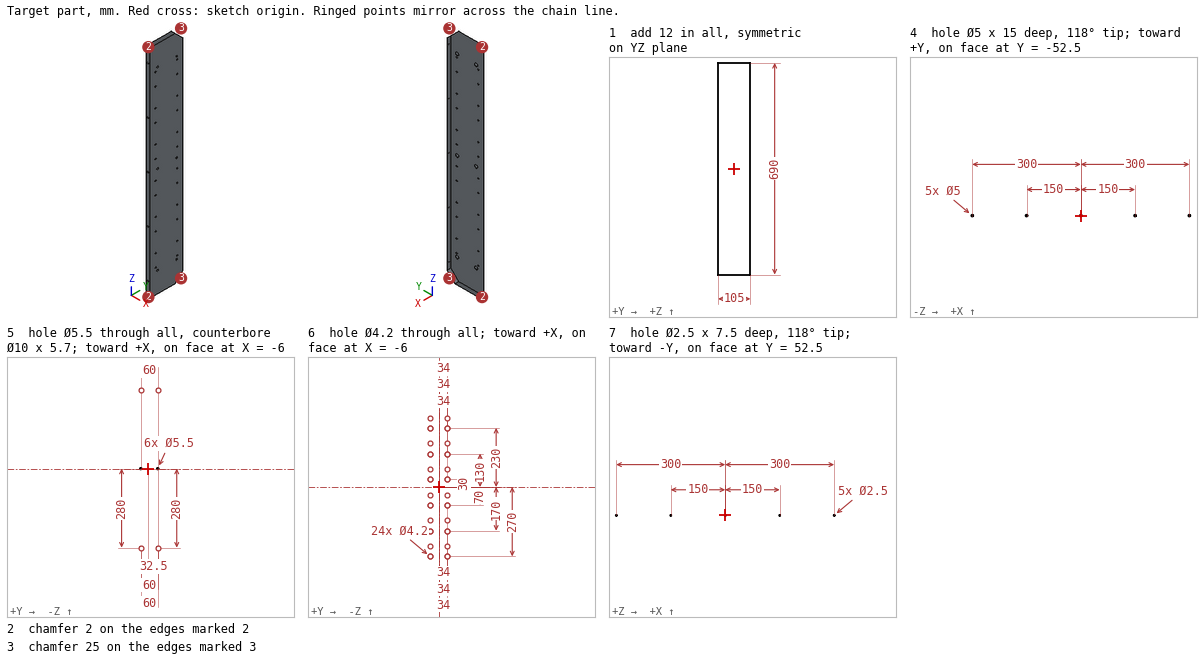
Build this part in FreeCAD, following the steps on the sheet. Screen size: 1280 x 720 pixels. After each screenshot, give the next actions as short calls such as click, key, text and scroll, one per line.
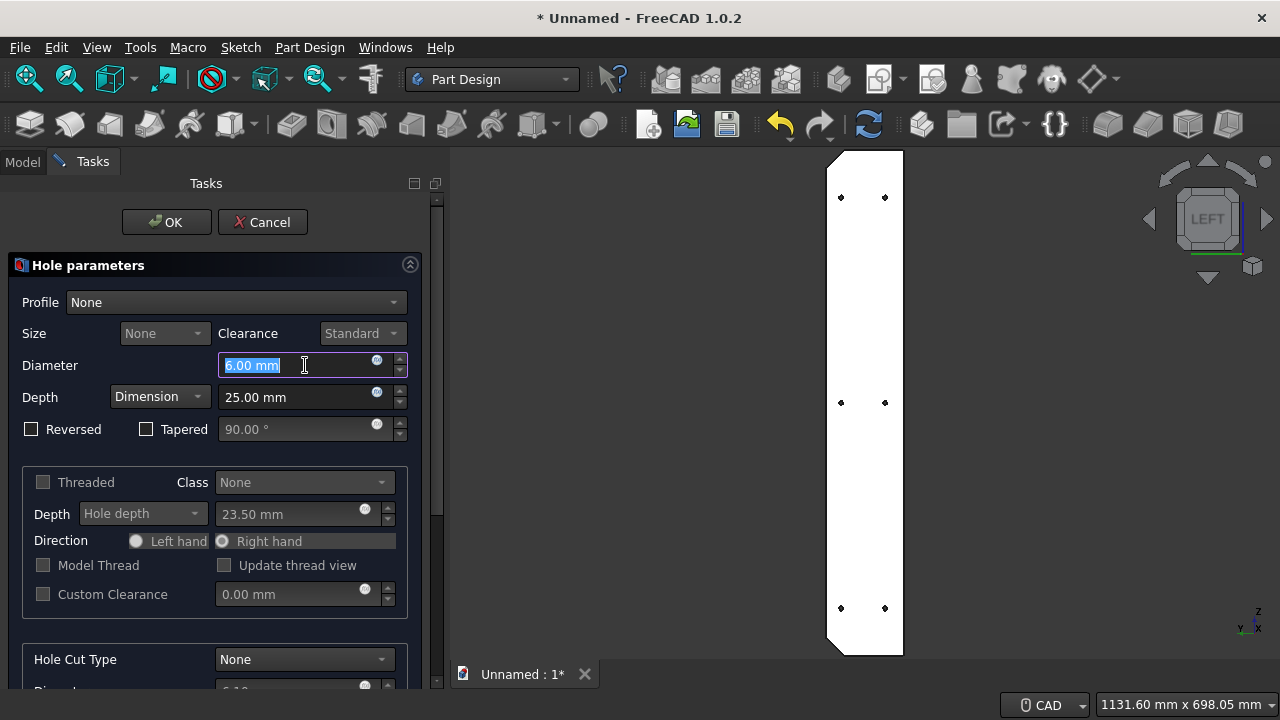
text(5.5)
key(Tab)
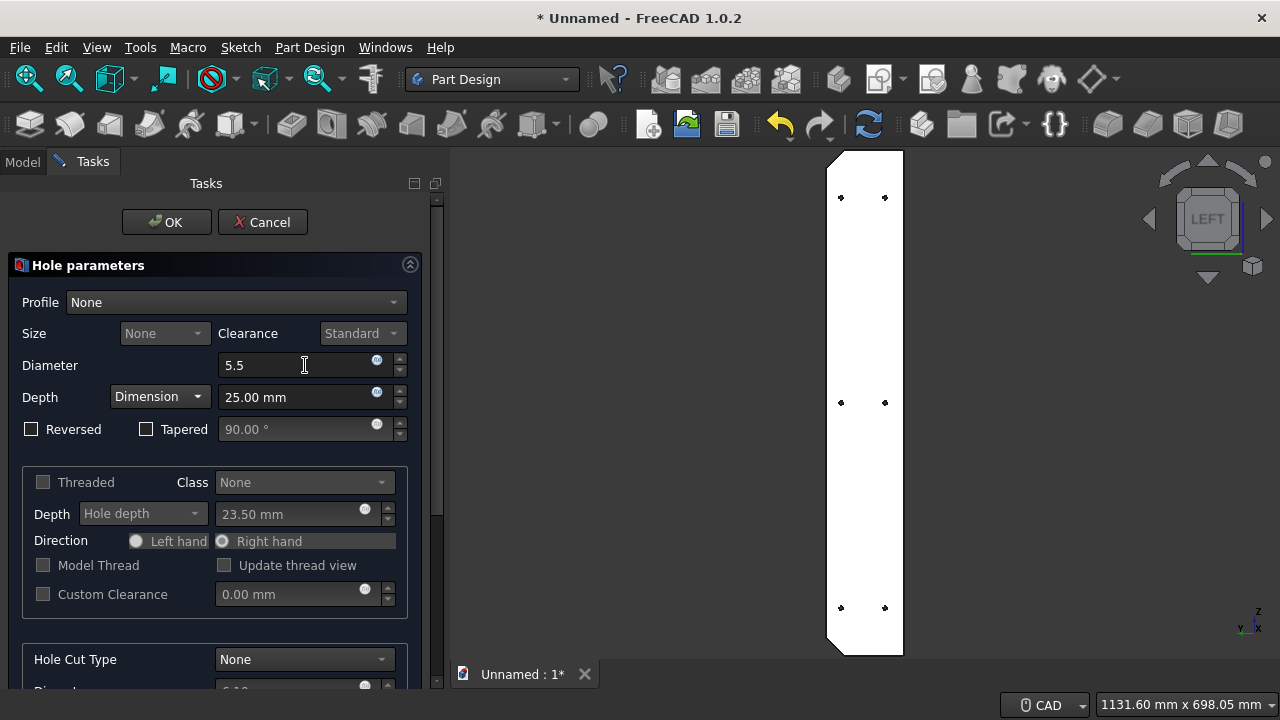
click(161, 396)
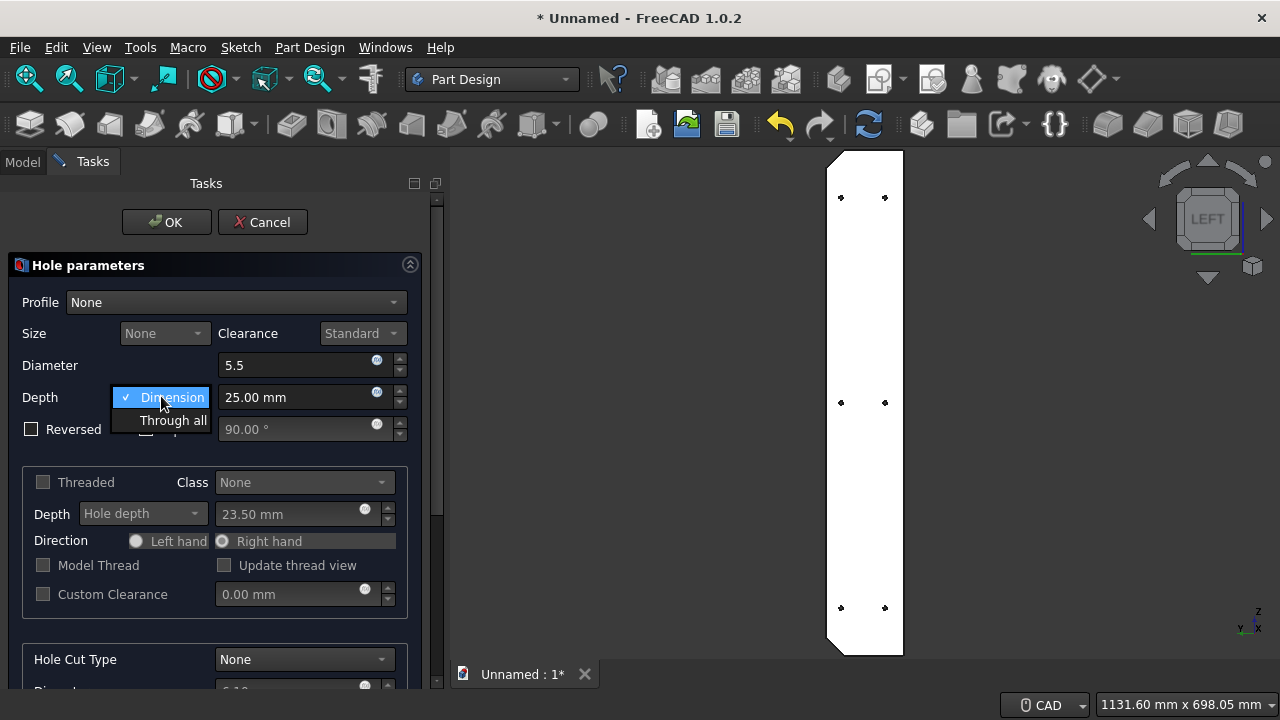
click(160, 420)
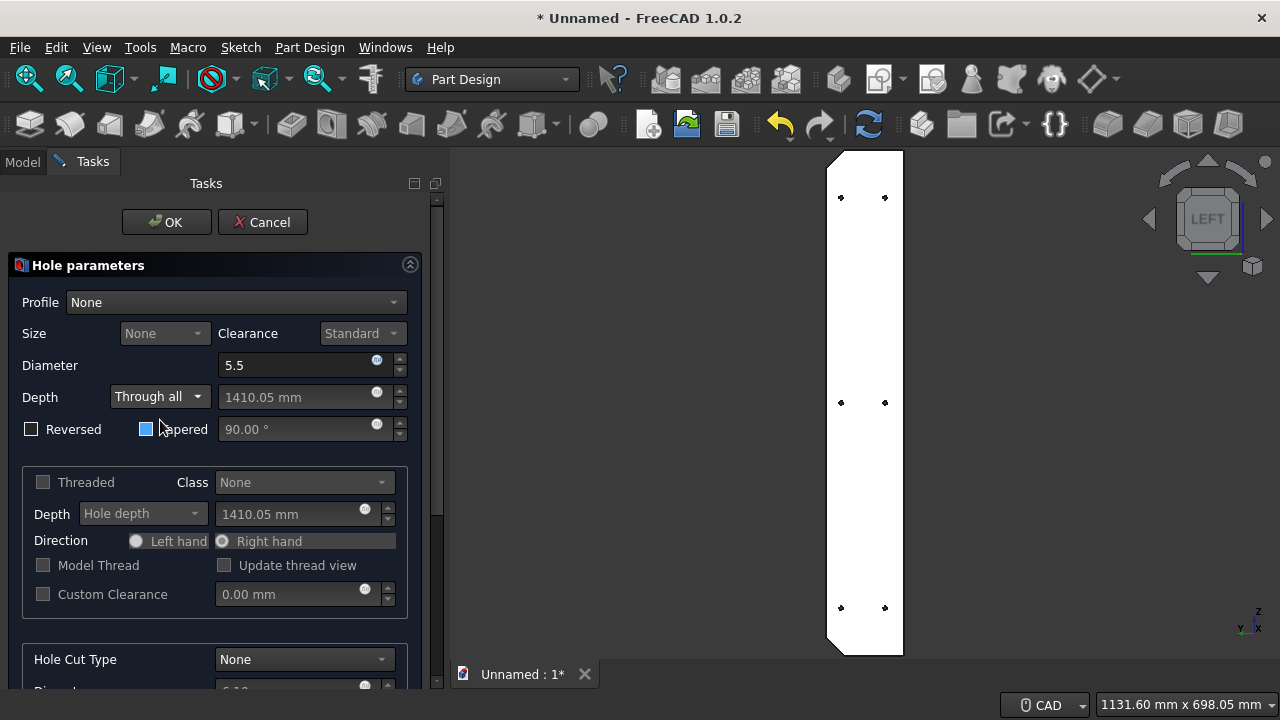
click(306, 660)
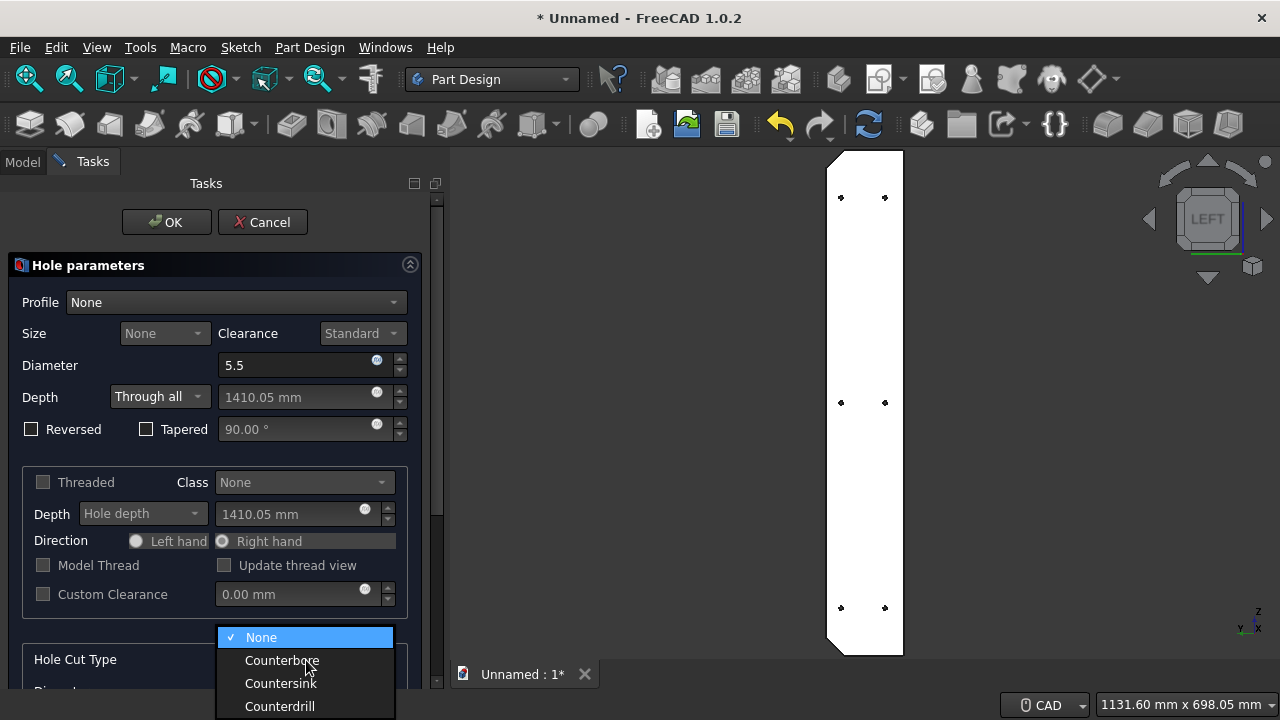
click(304, 660)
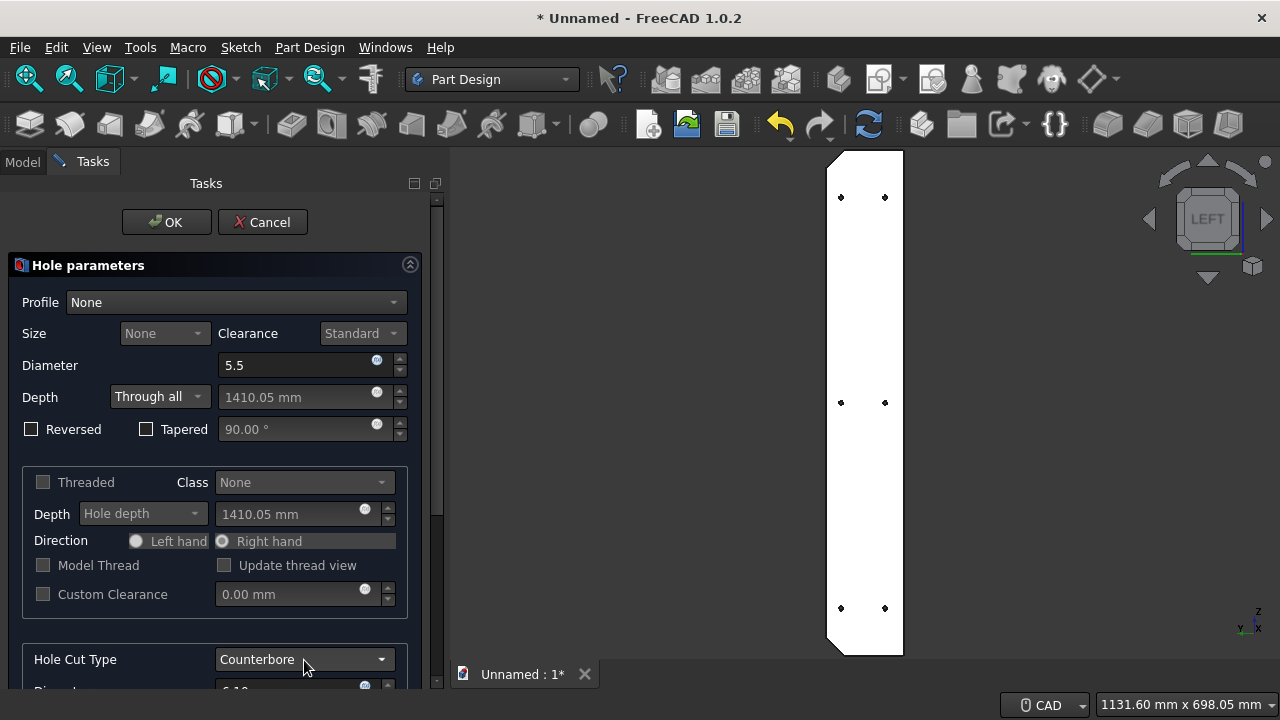
scroll(437, 440, down, 2)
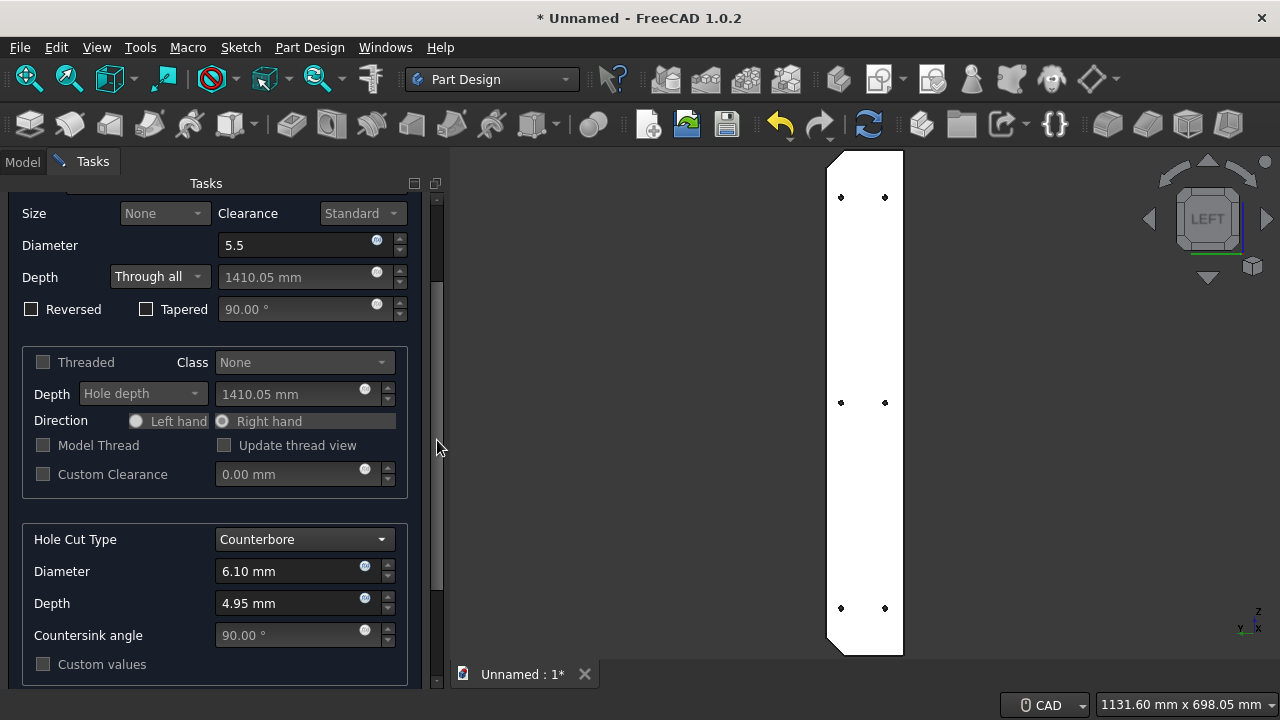
triple_click(298, 571)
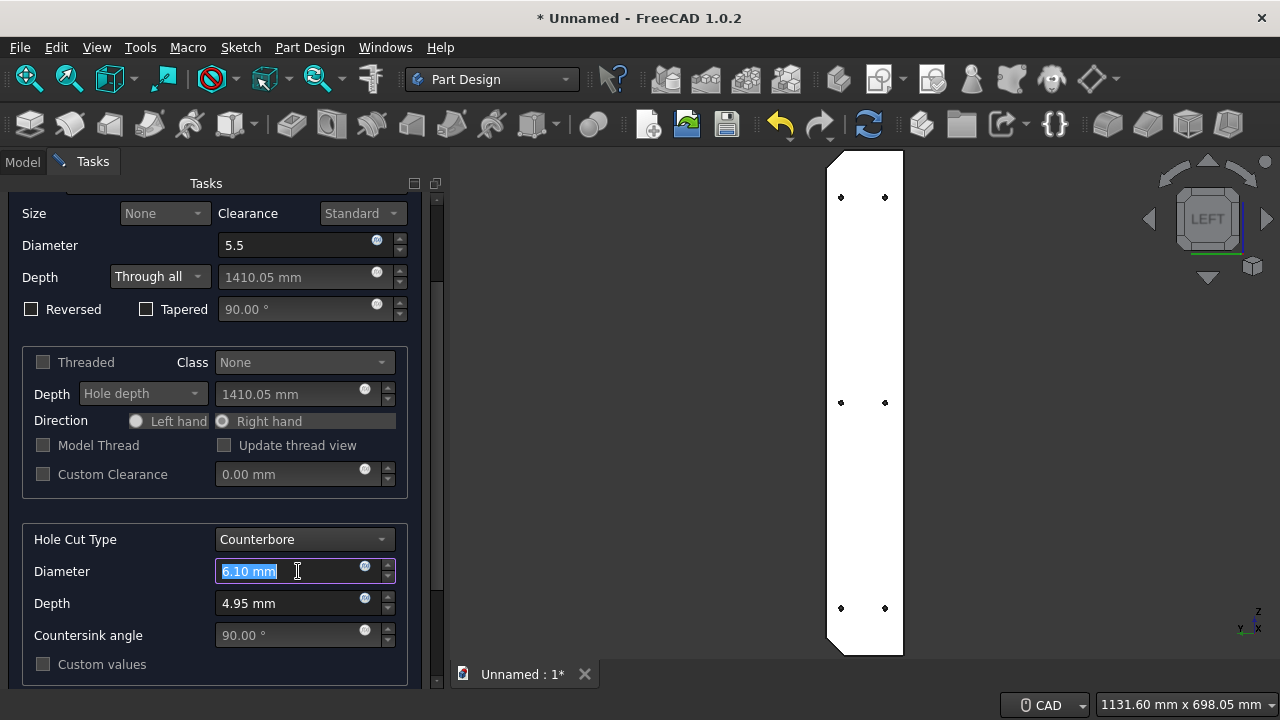
text(10)
key(Tab)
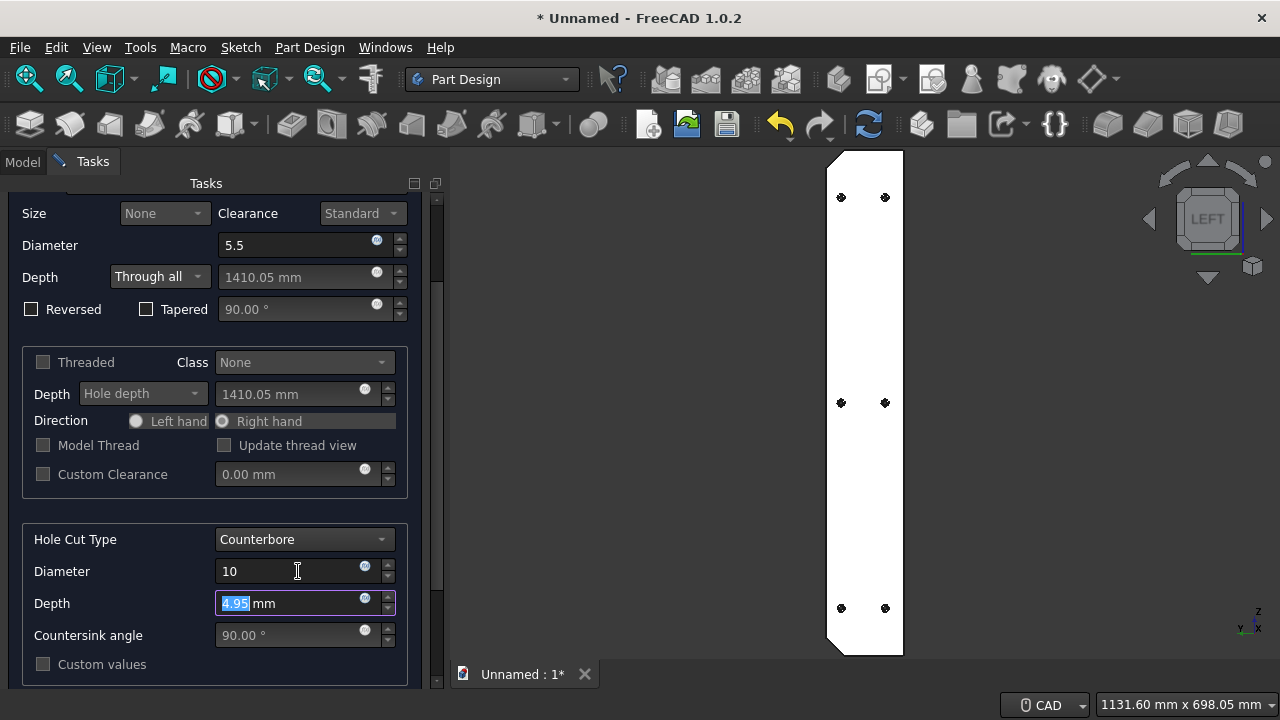
text(5.7)
key(Tab)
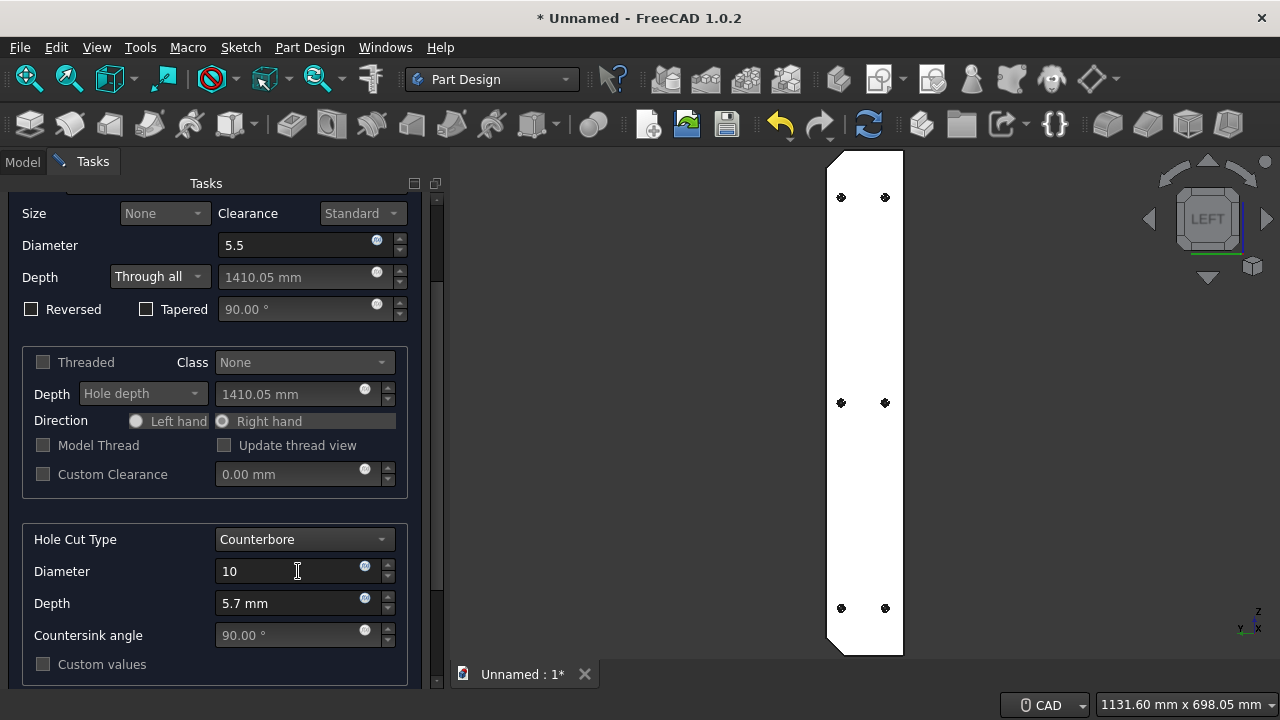
scroll(437, 440, up, 3)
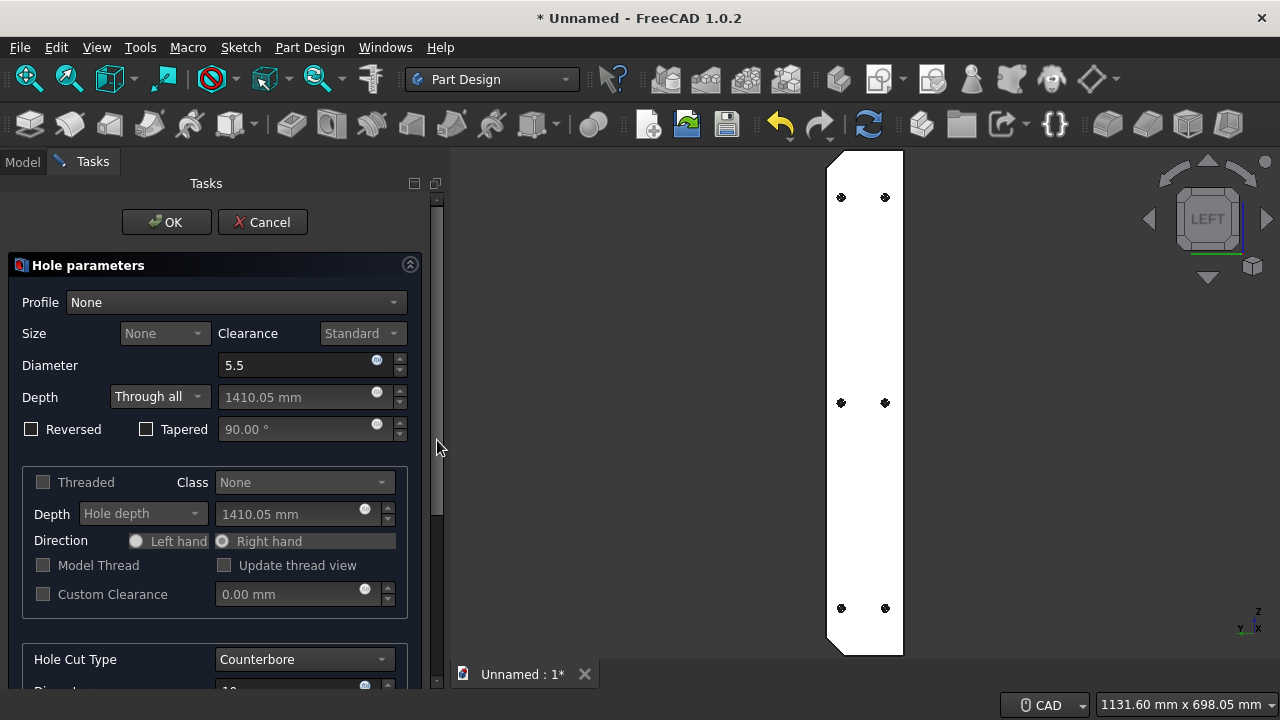
click(167, 222)